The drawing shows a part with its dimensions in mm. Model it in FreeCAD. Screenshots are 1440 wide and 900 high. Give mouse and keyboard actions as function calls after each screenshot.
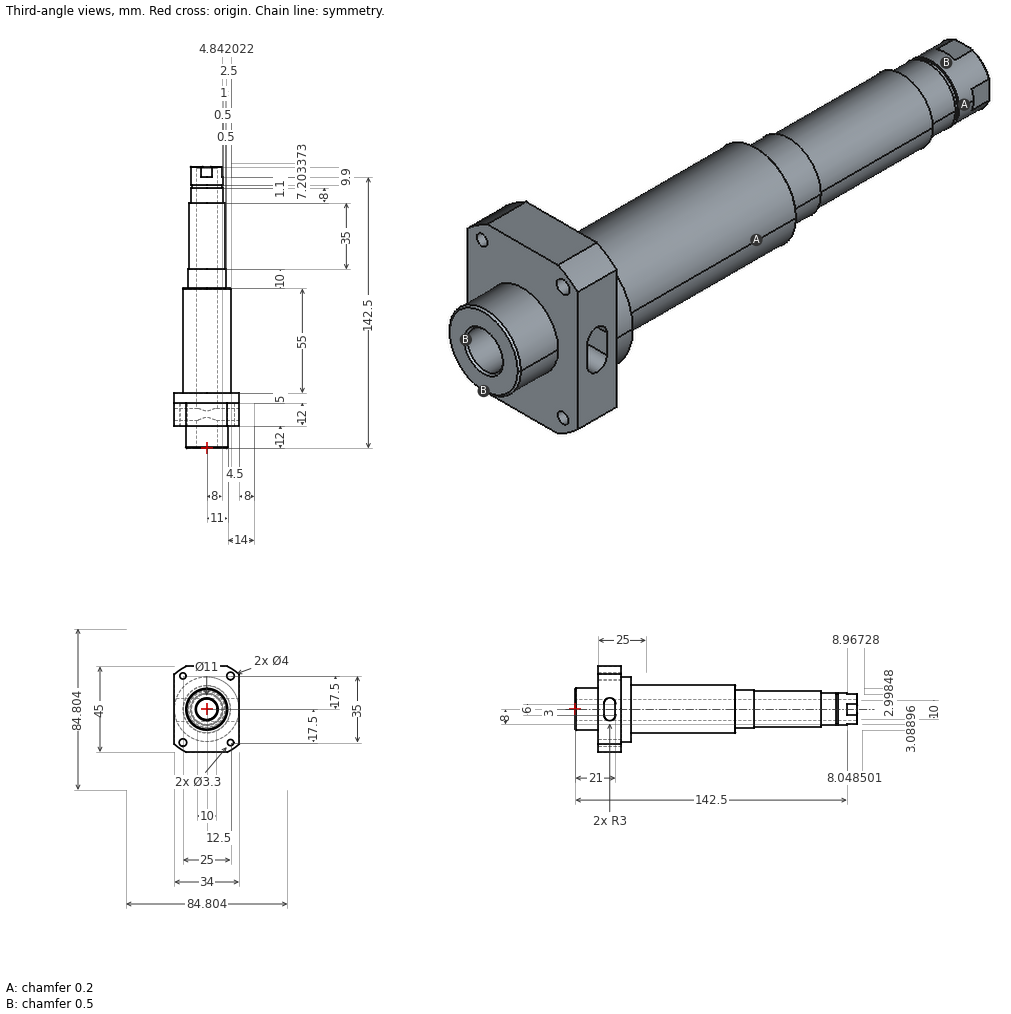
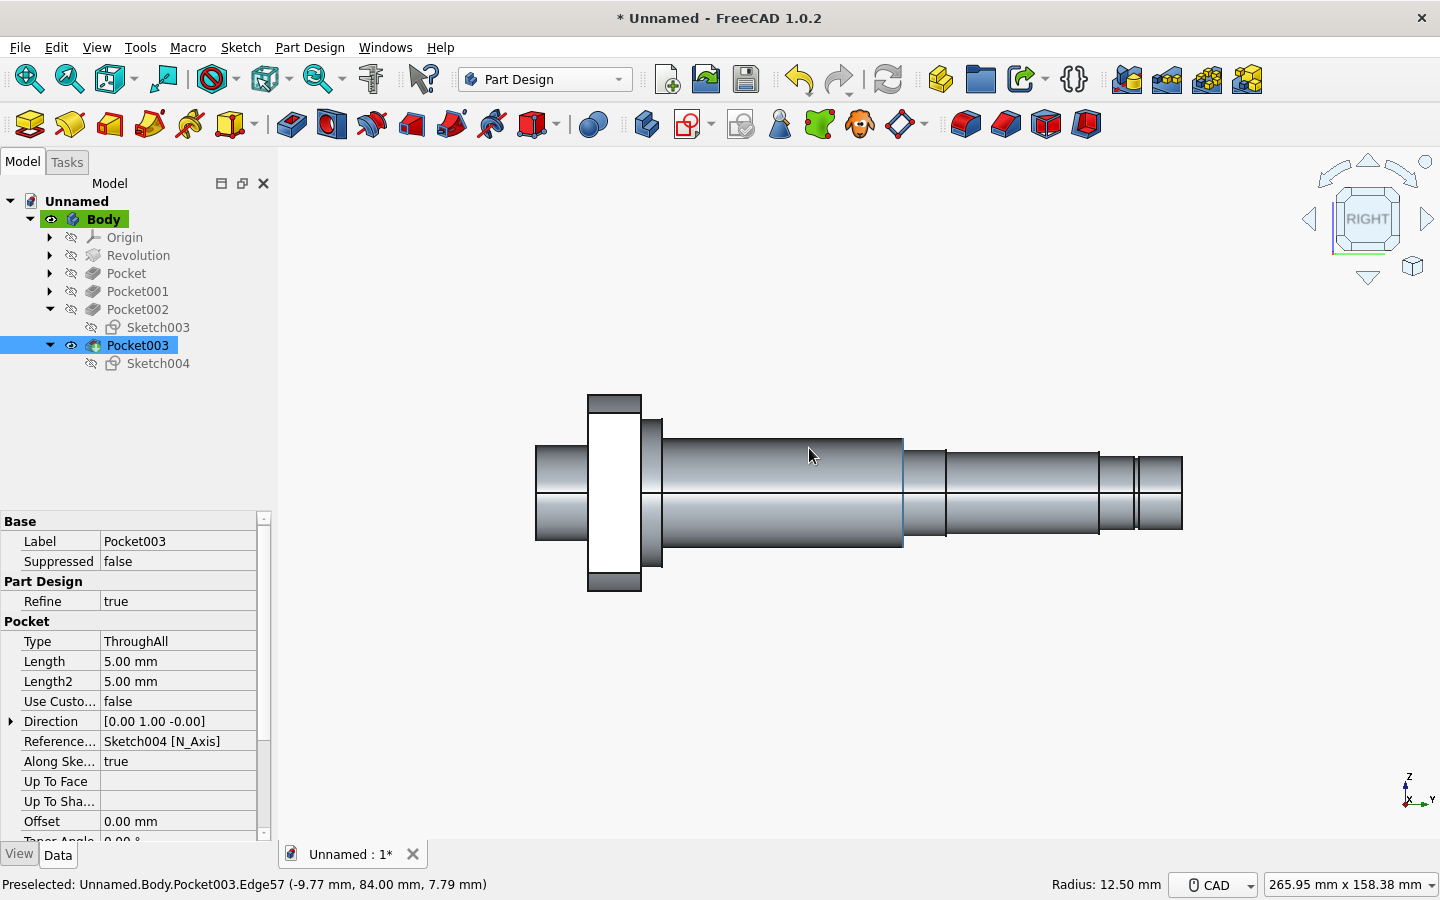
click(1182, 470, ctrl)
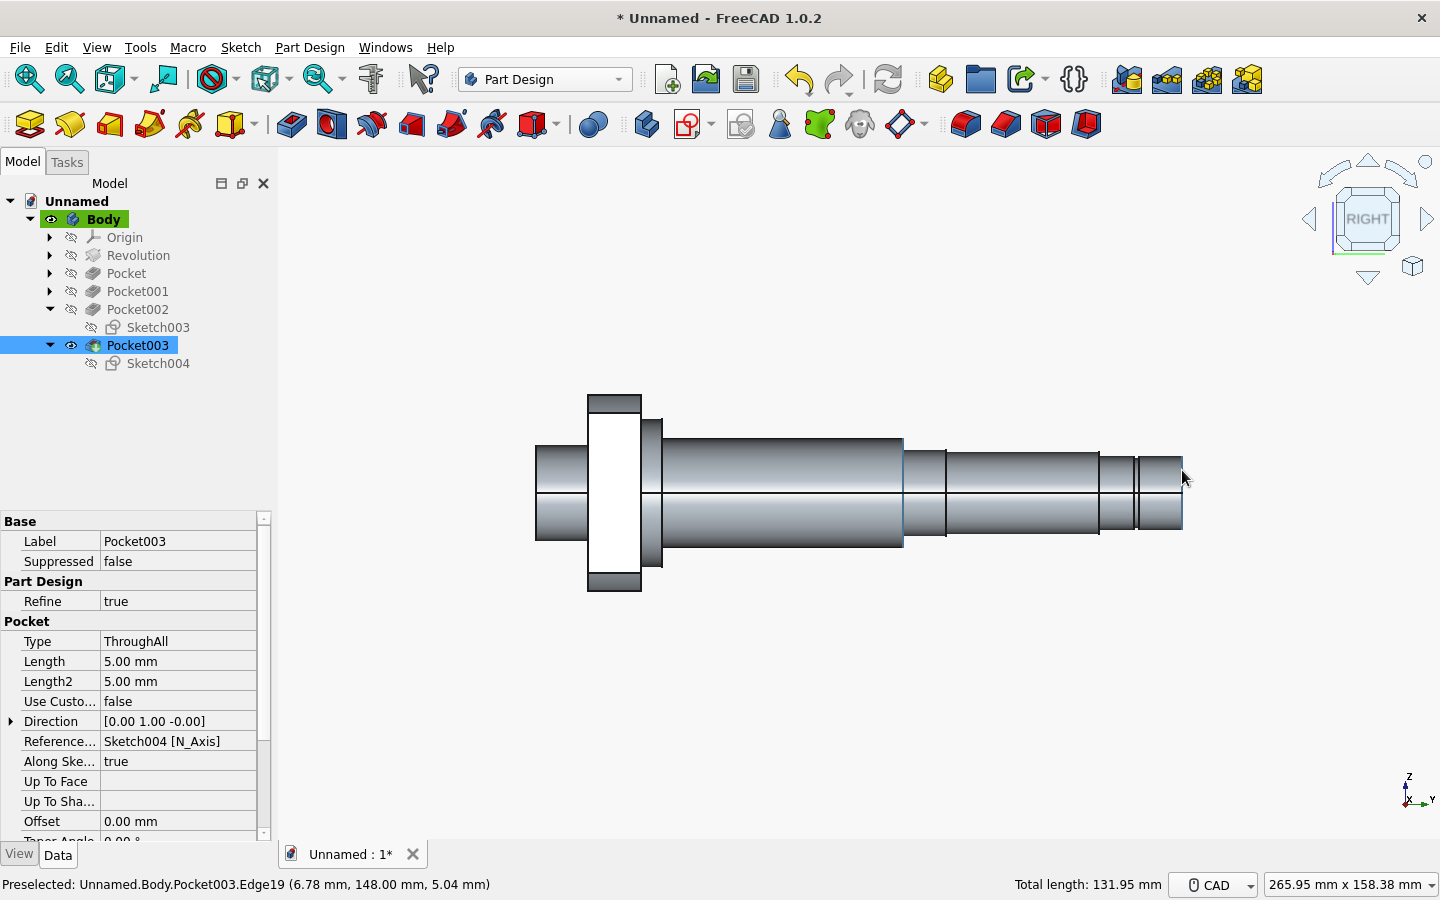
click(1006, 124)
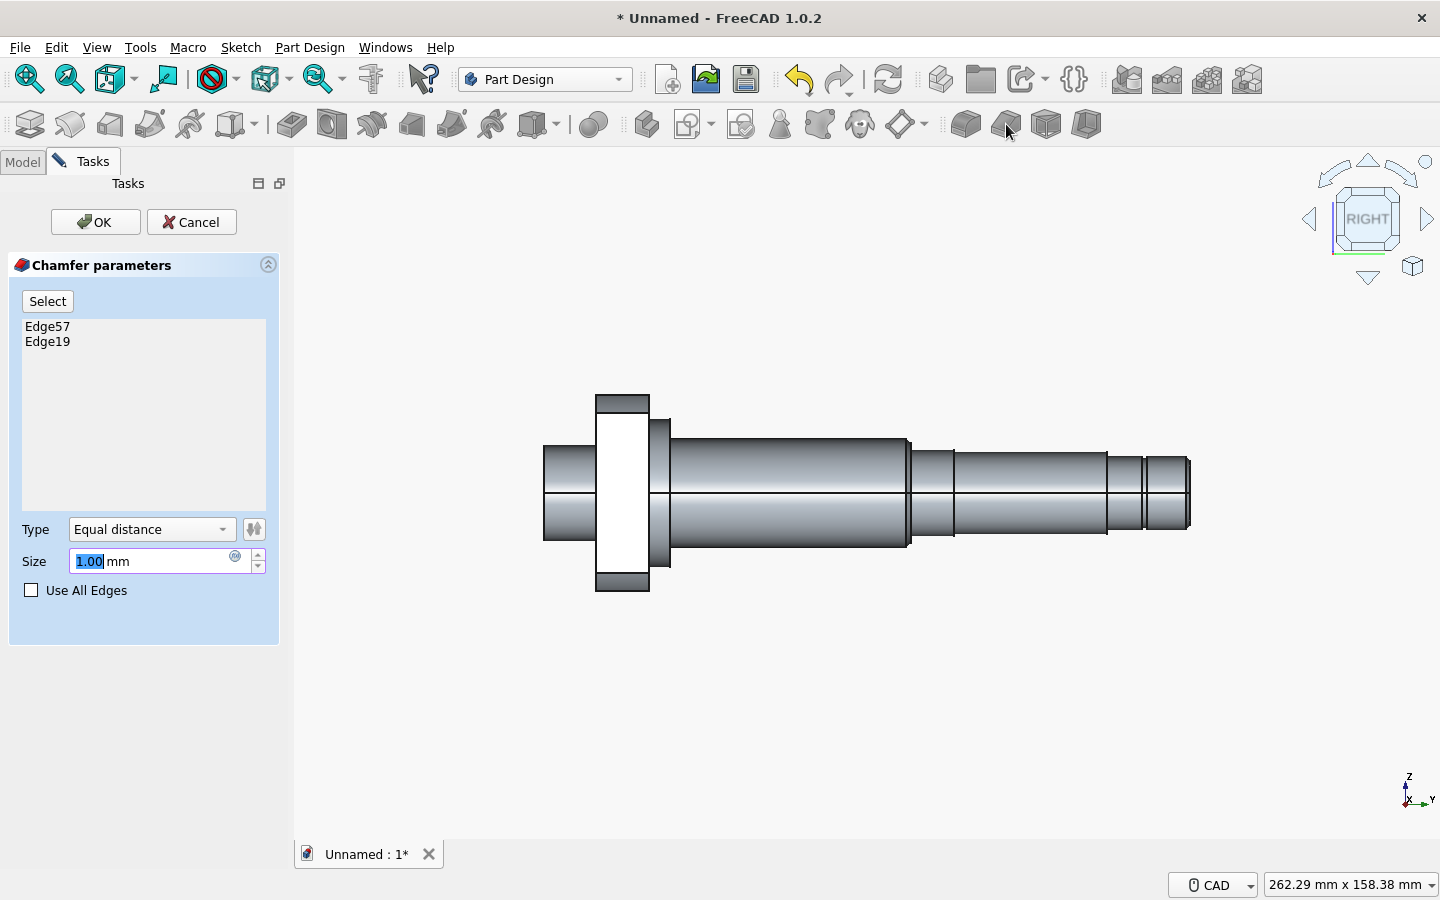
text(0.2)
key(Tab)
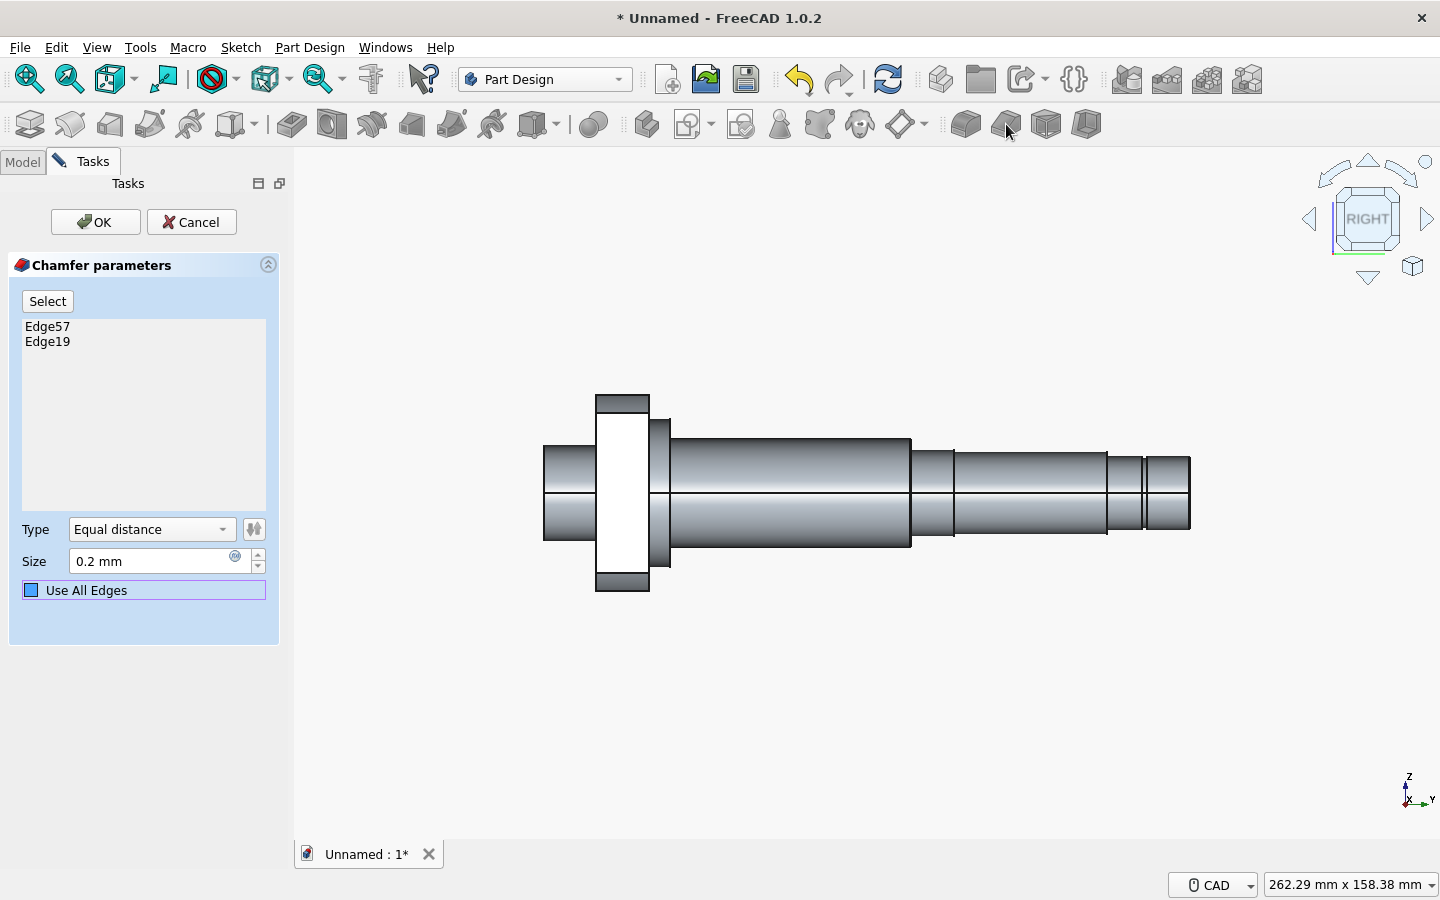
click(96, 222)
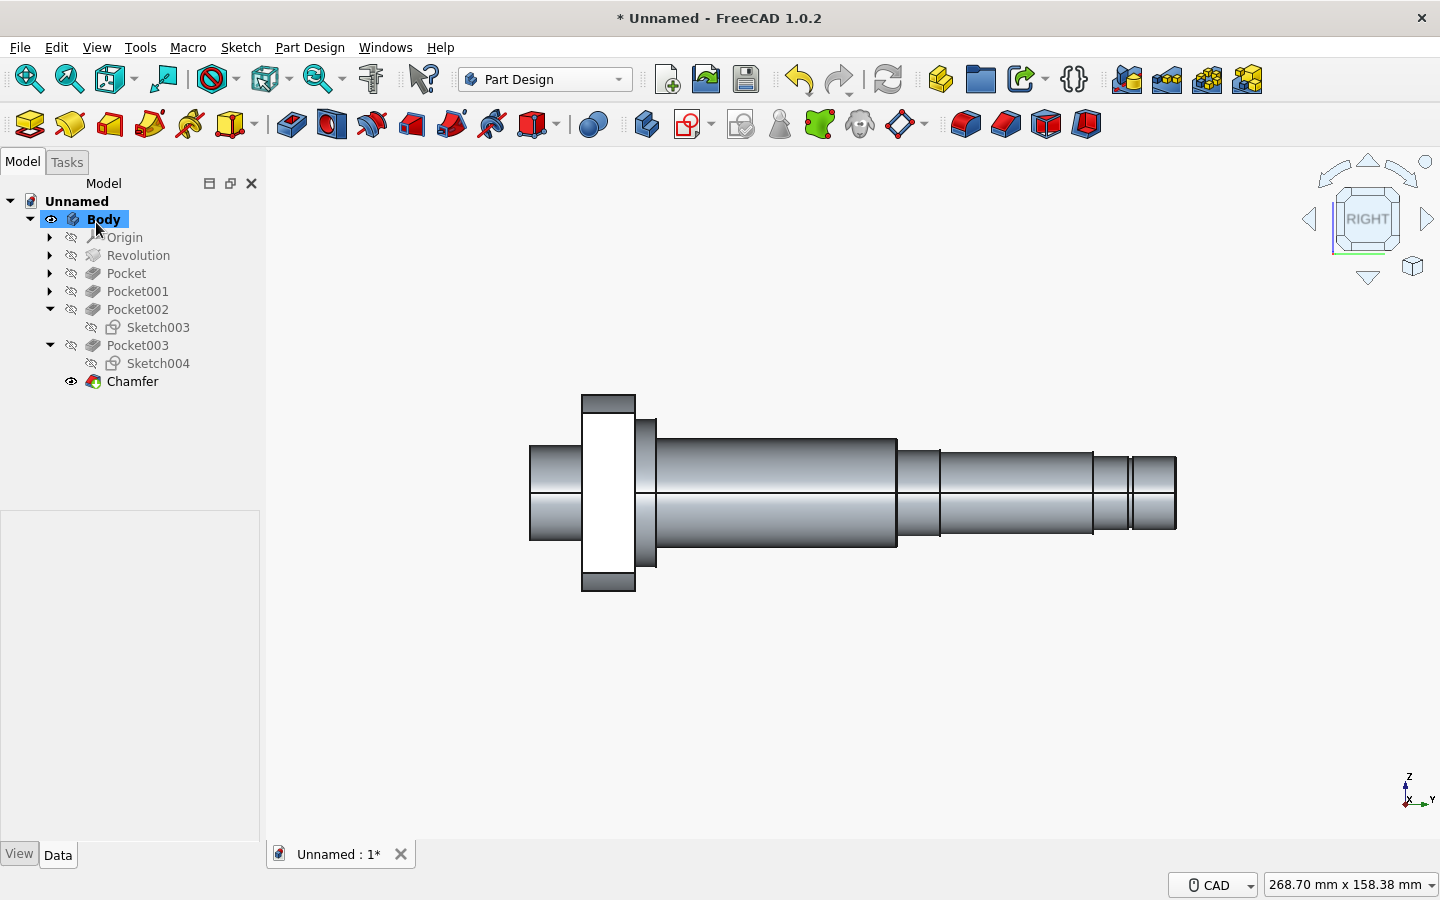
click(530, 464)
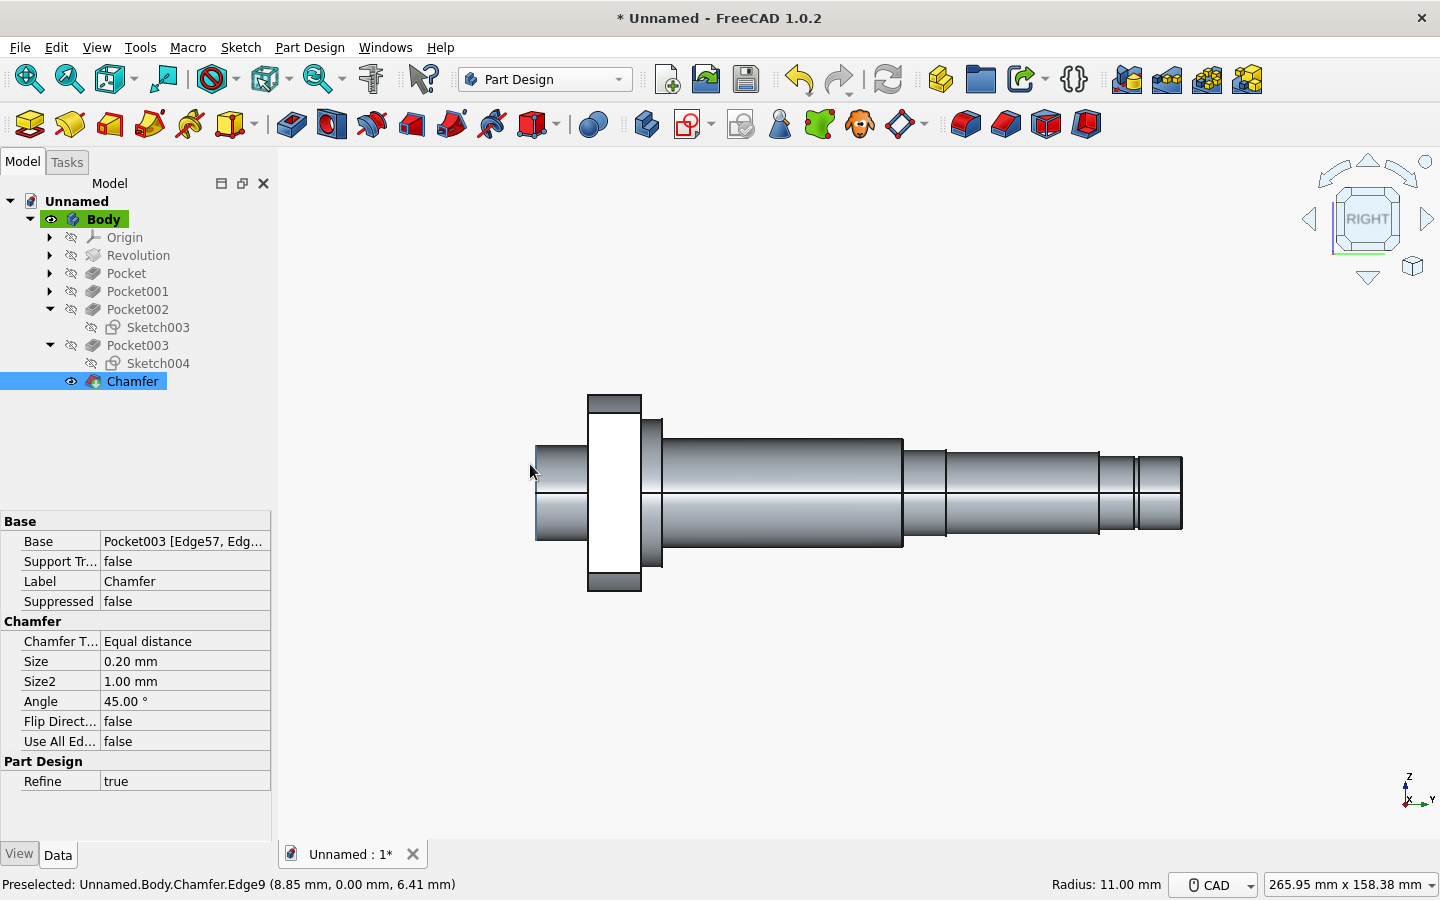
key(0)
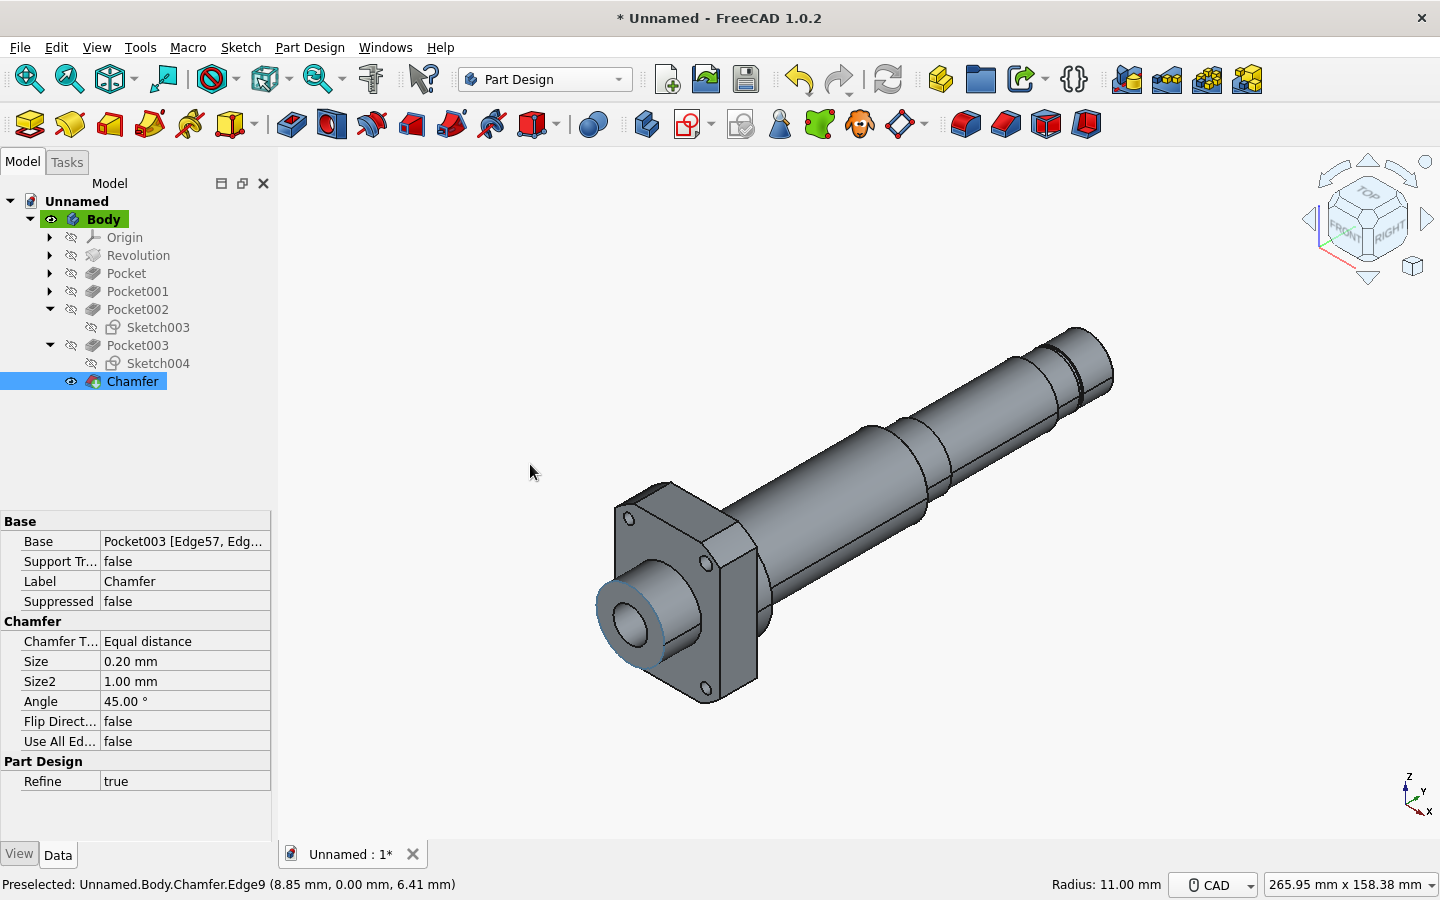
click(613, 614, ctrl)